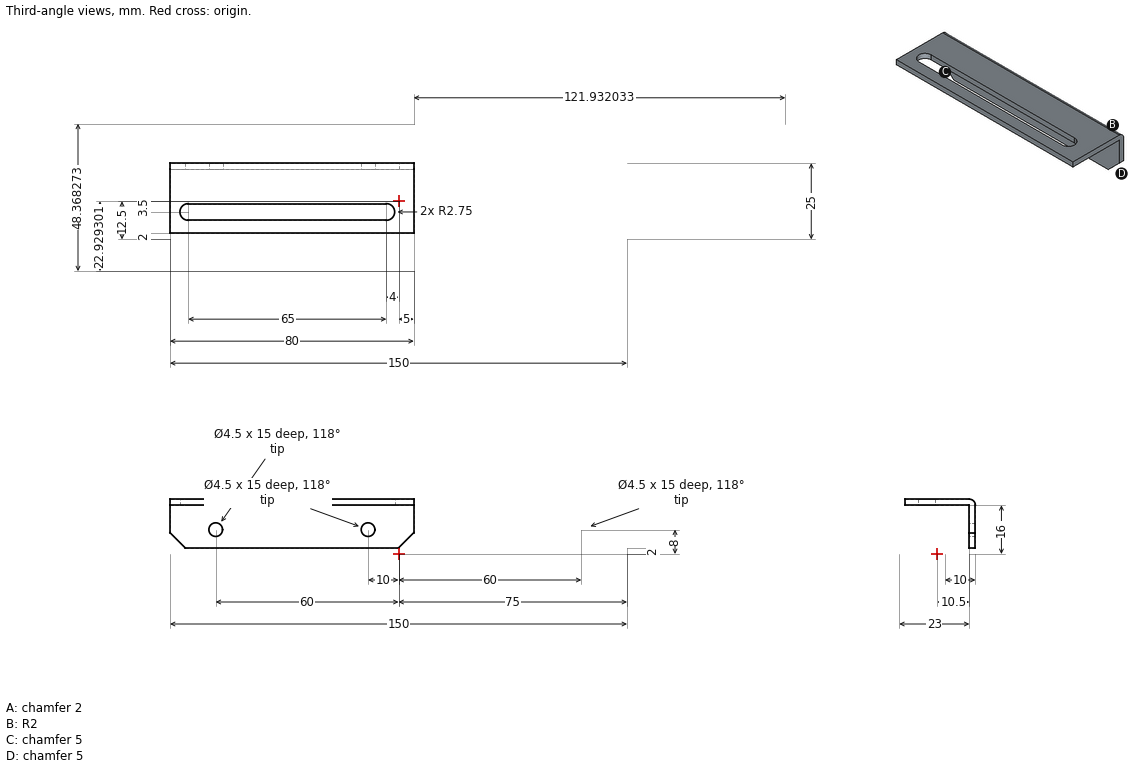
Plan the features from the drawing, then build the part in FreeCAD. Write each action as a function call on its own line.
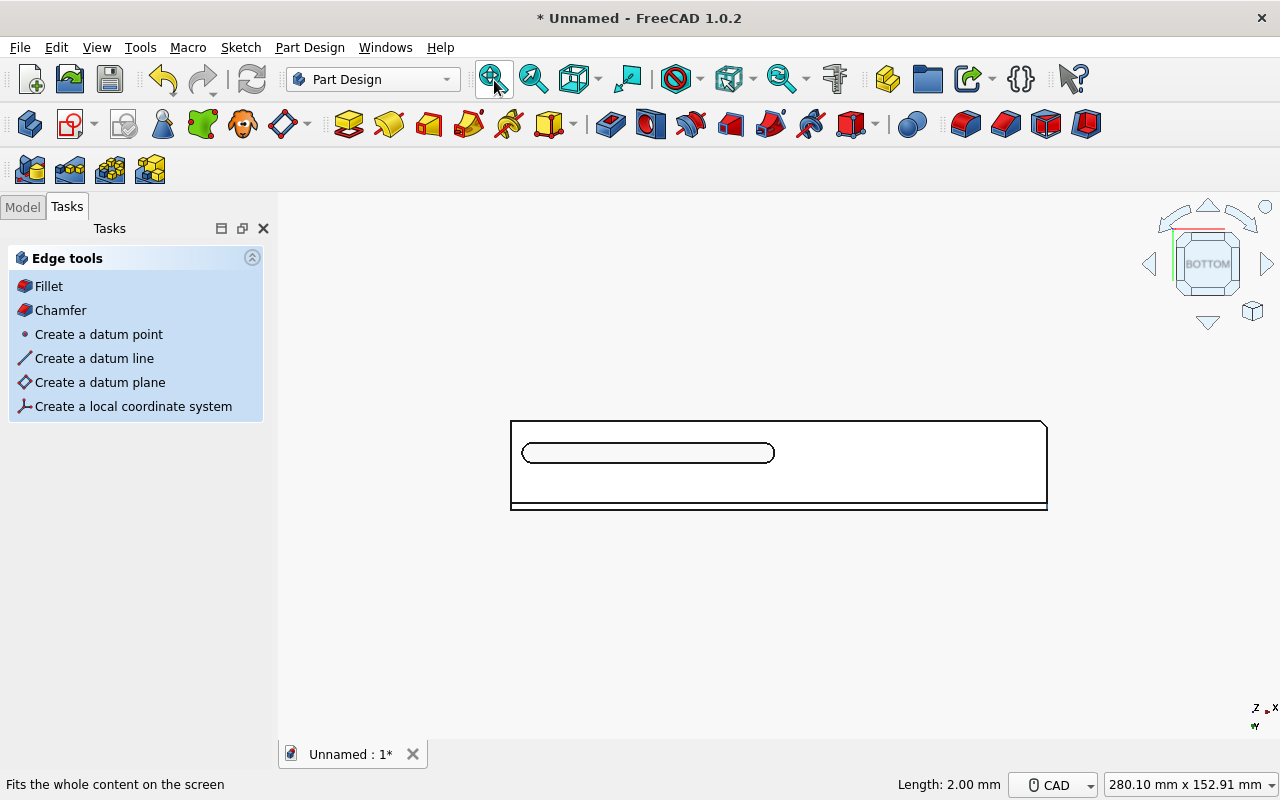
scroll(511, 506, up, 9)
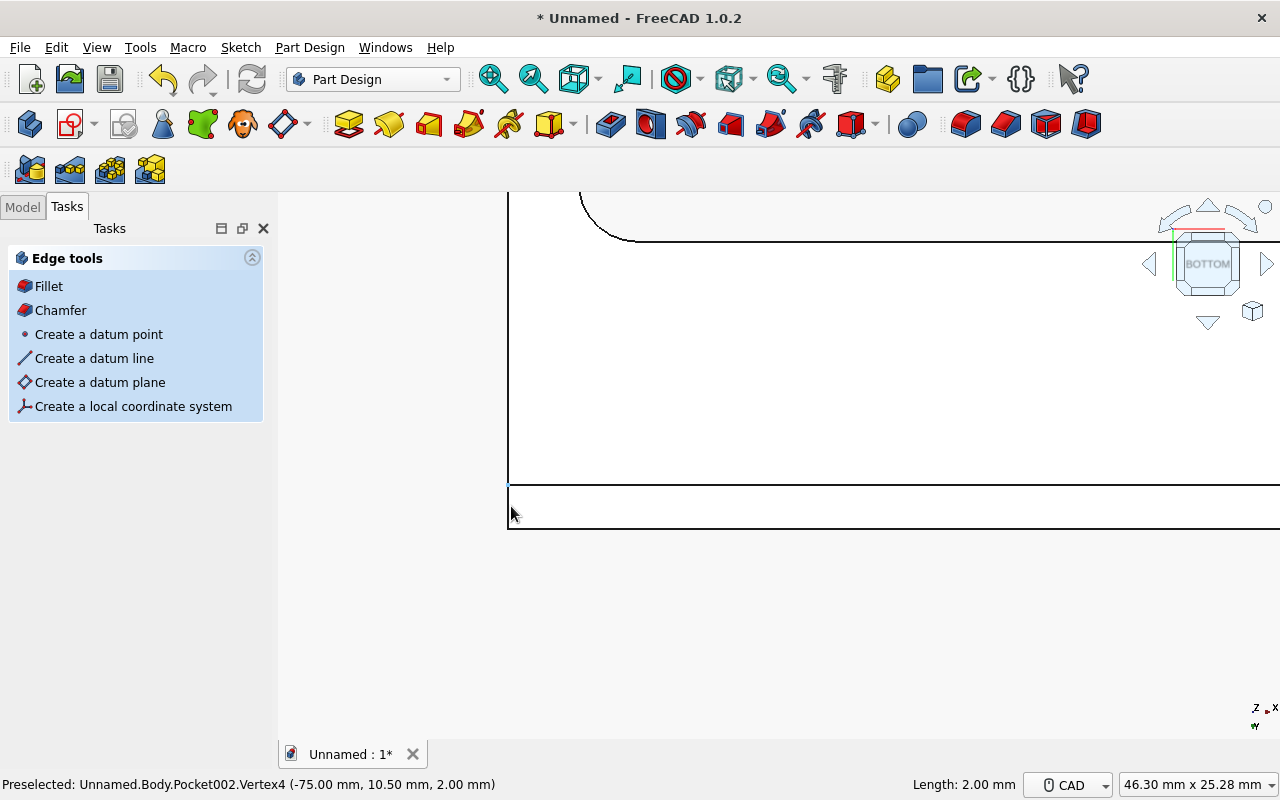
click(508, 506, ctrl)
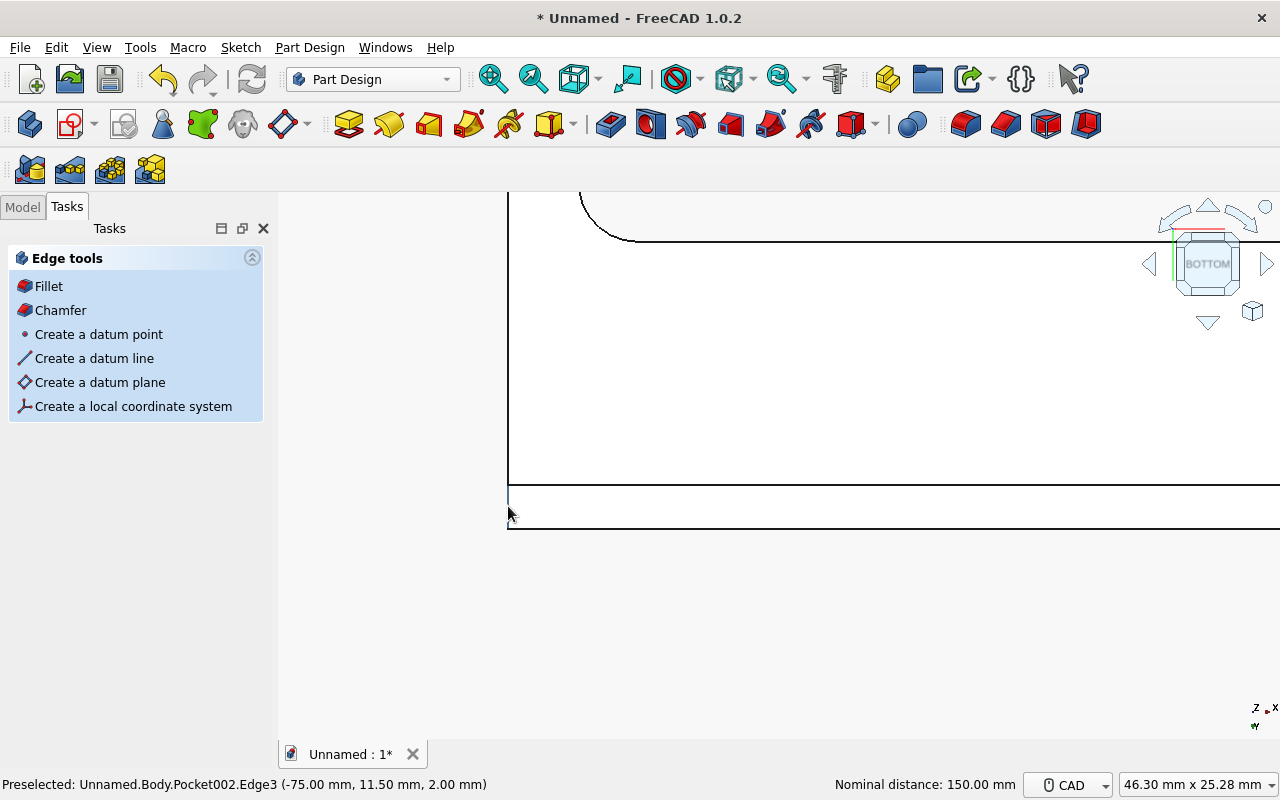
click(1006, 124)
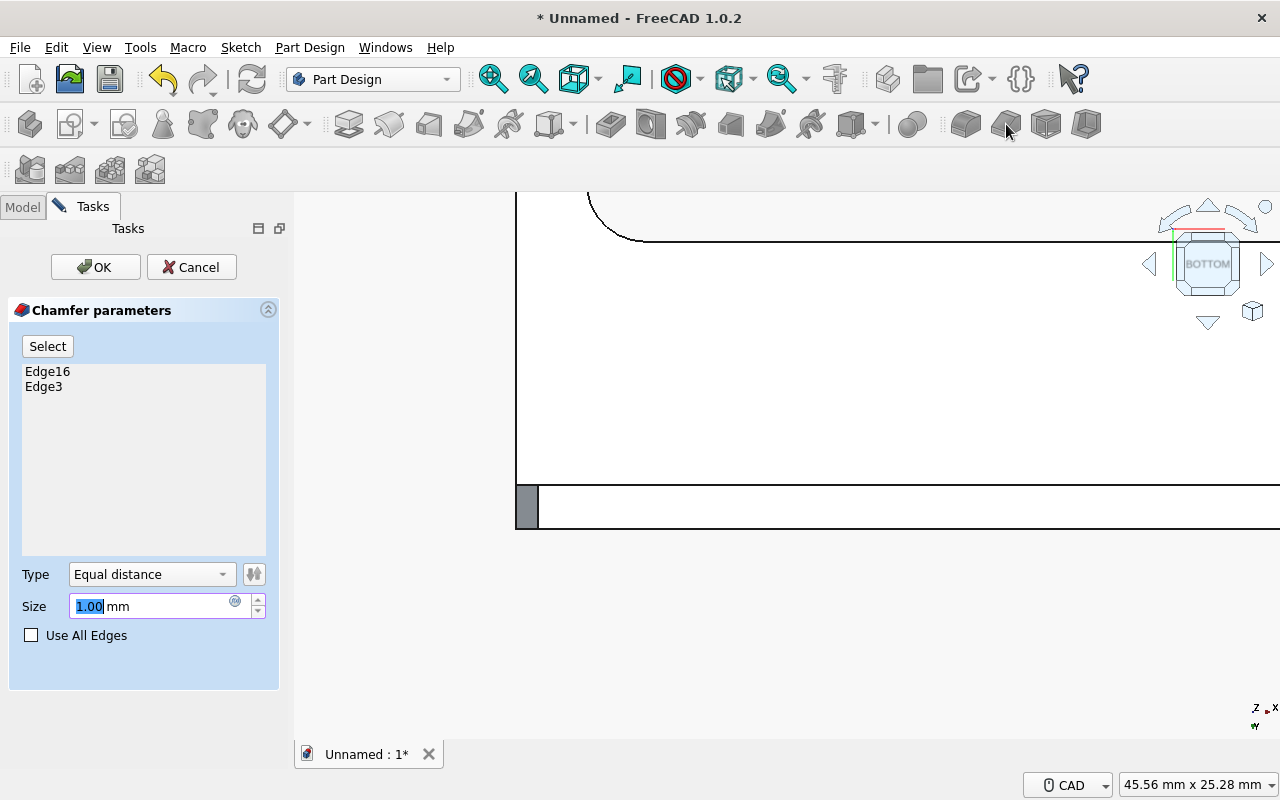
text(5)
key(Tab)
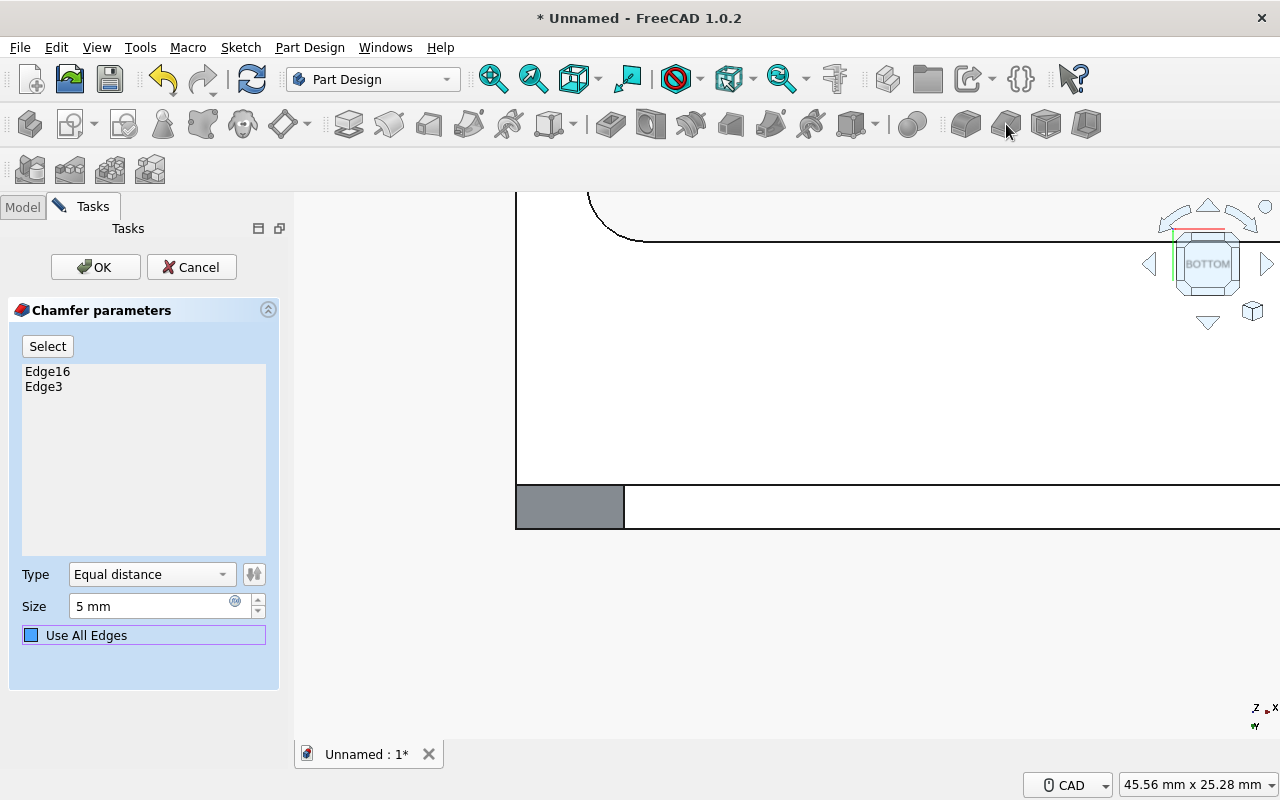
click(96, 267)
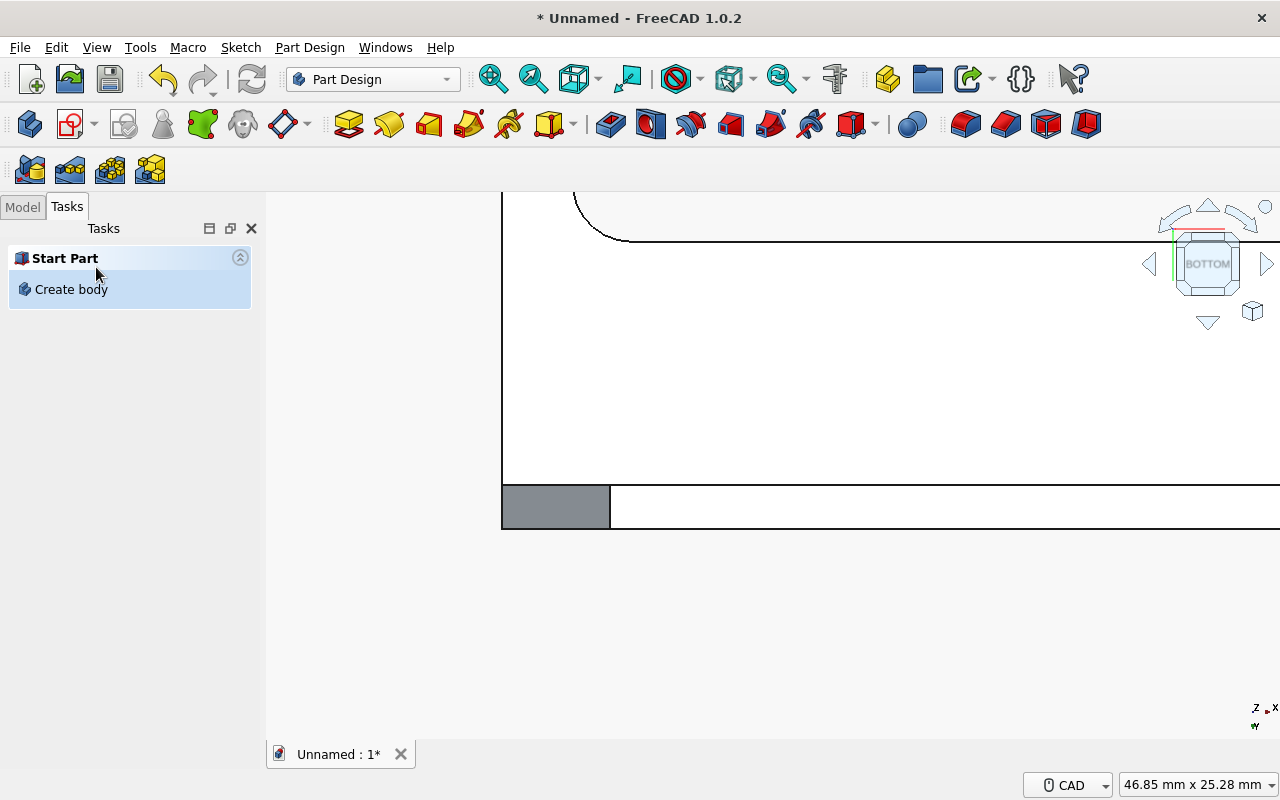
click(494, 80)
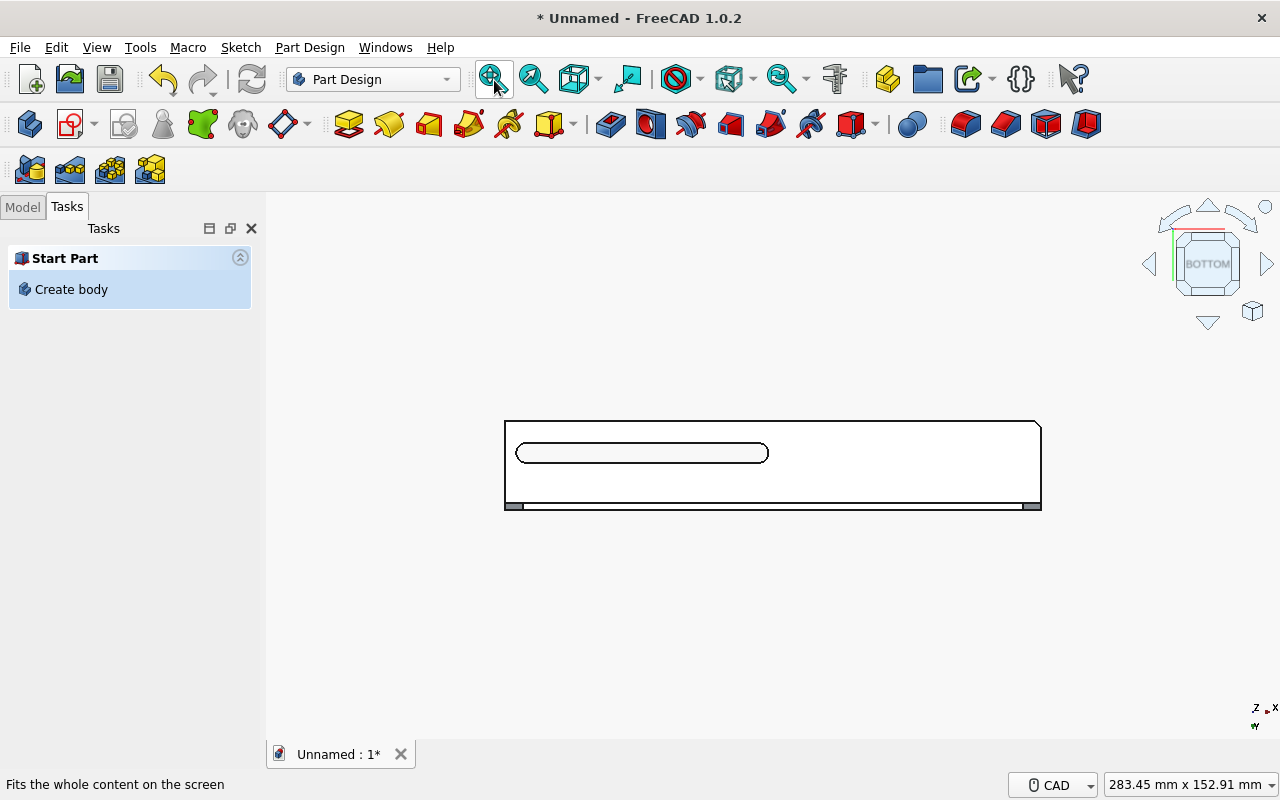
scroll(988, 506, up, 7)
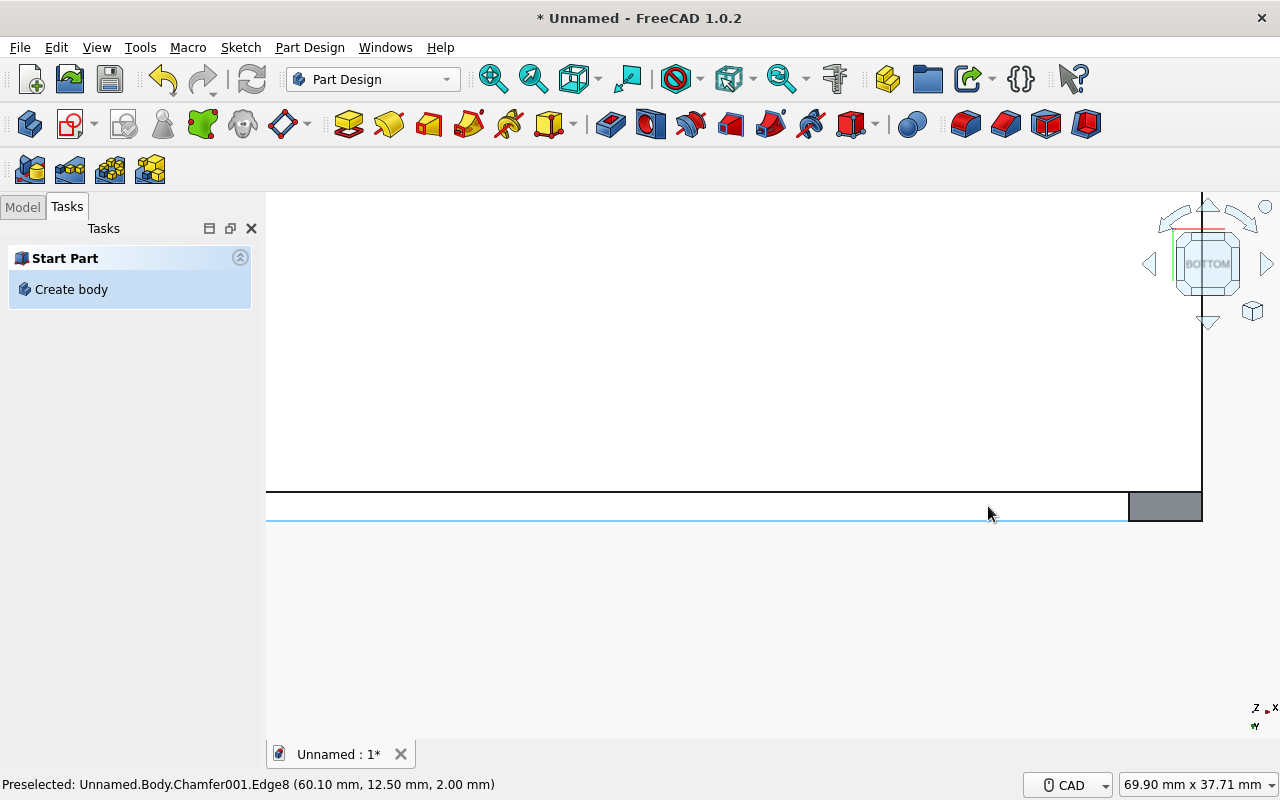
click(984, 506)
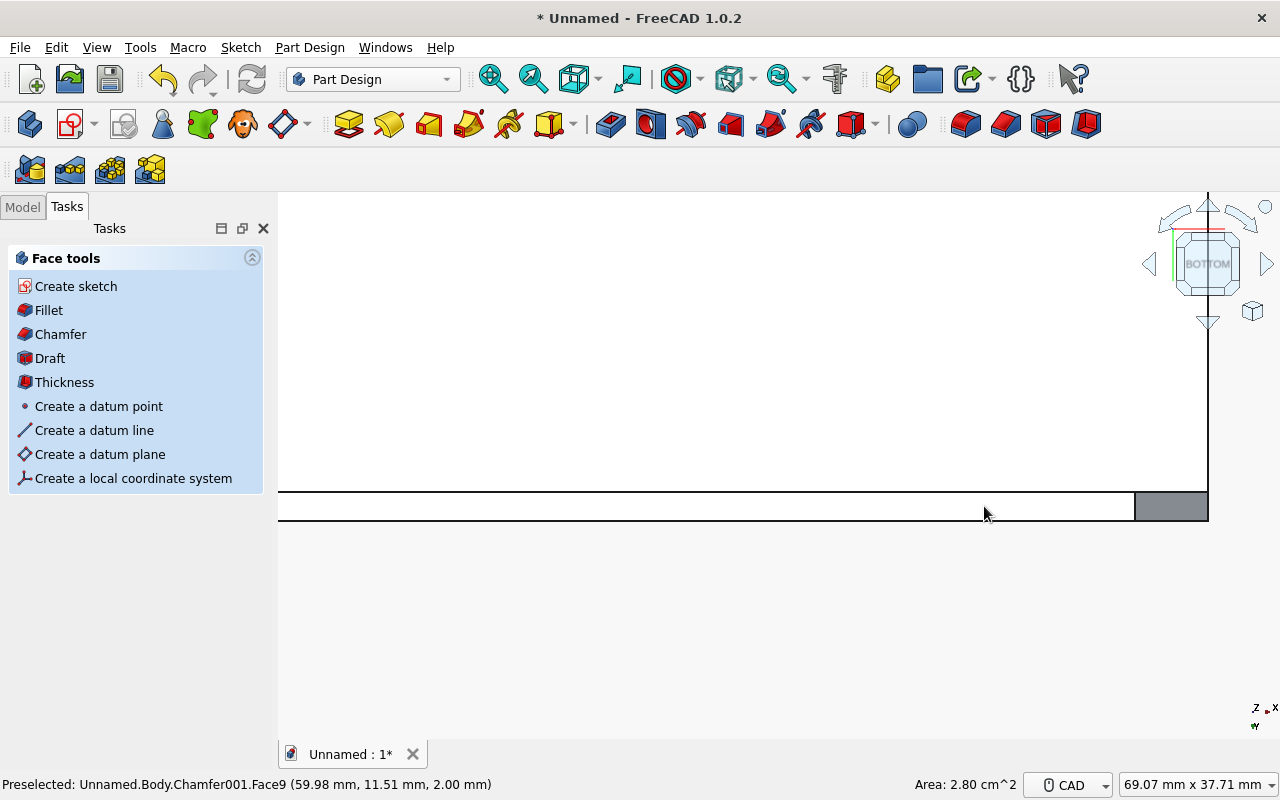
click(70, 124)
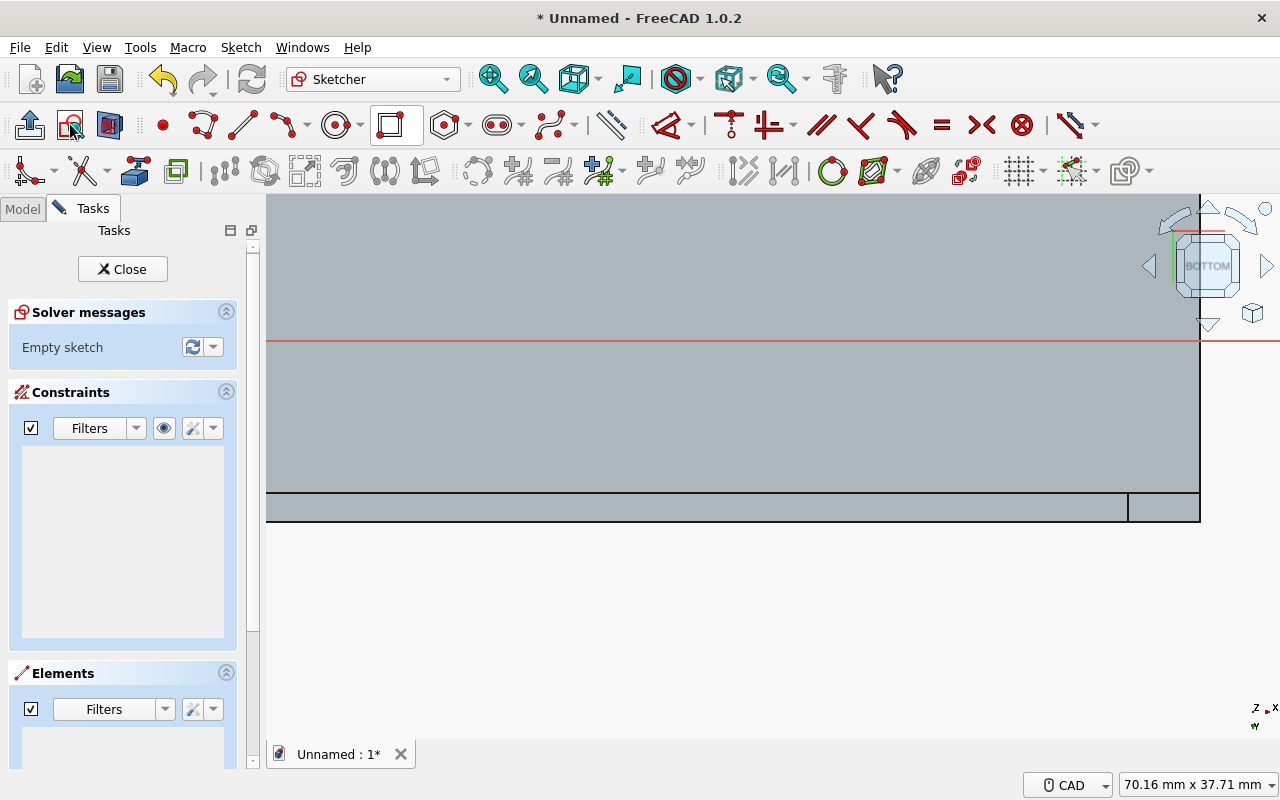
scroll(563, 513, down, 6)